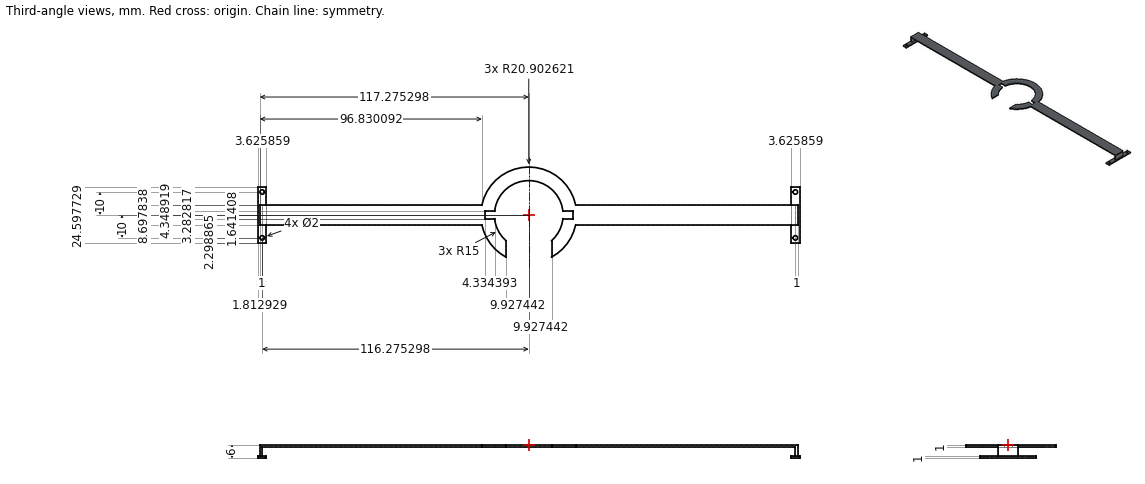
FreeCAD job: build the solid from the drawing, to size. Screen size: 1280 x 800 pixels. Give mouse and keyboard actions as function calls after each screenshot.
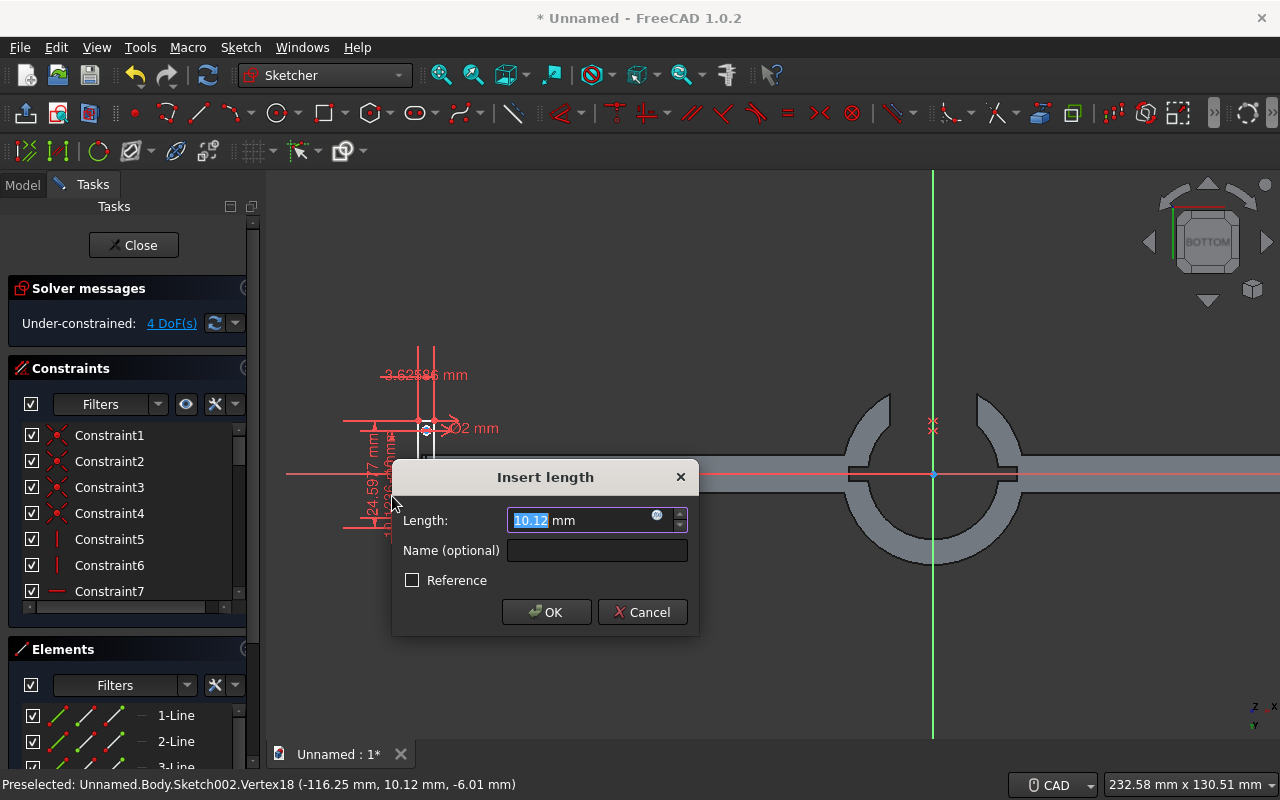
text(10)
key(Return)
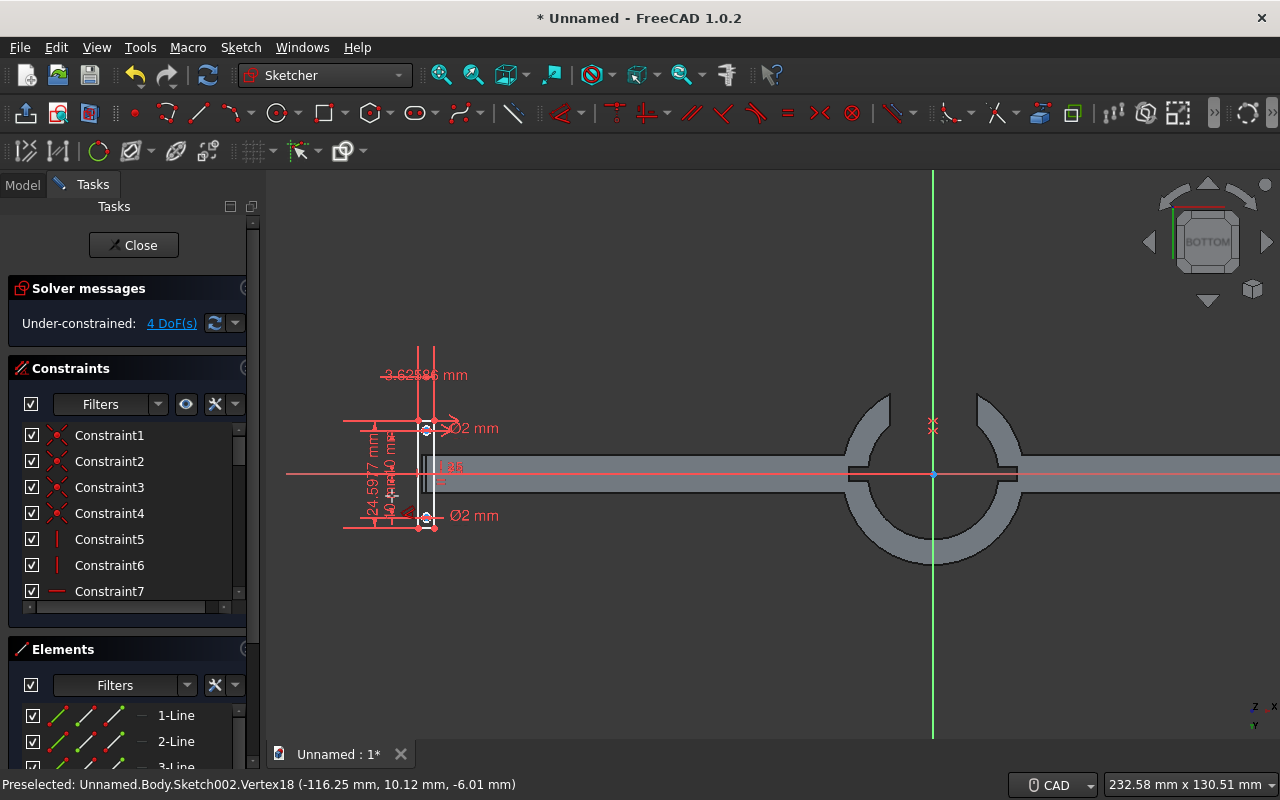
scroll(426, 431, down, 3)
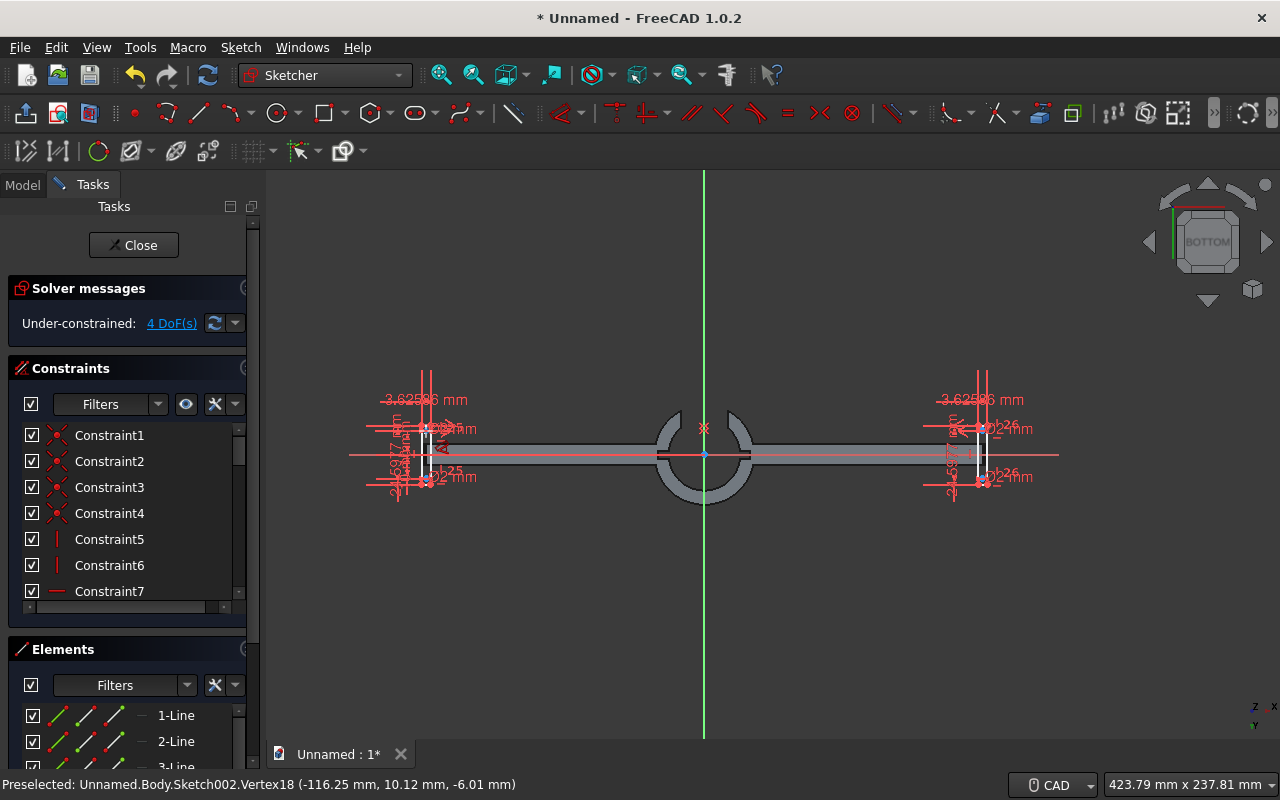
scroll(983, 479, up, 3)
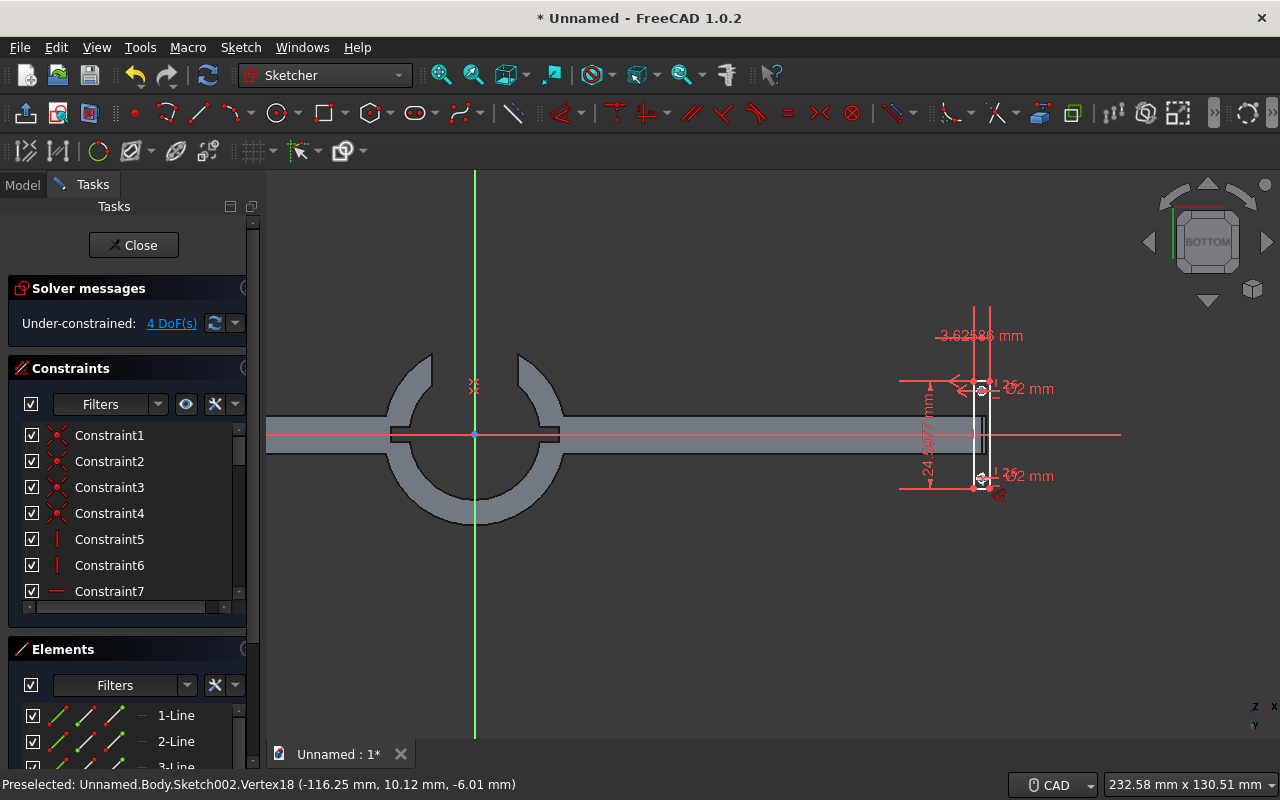
click(982, 478)
click(1016, 456)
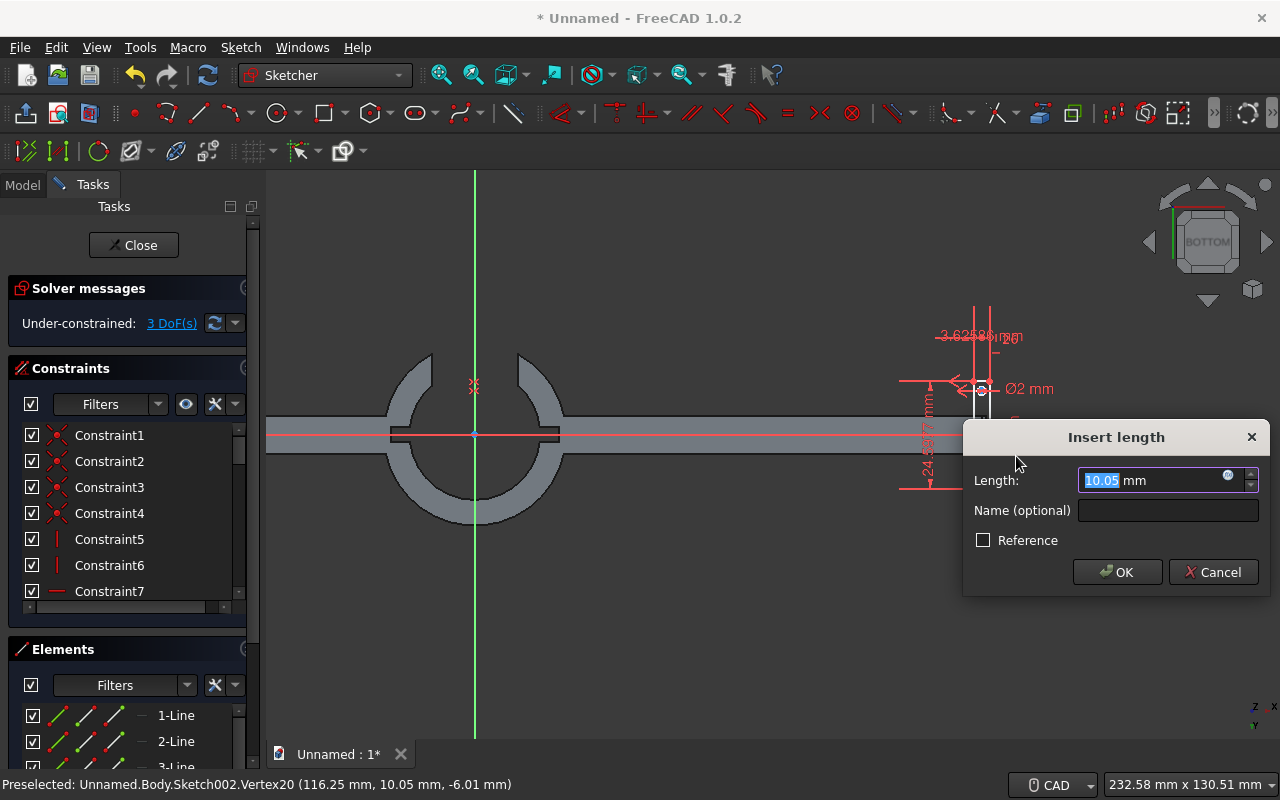
text(10)
key(Return)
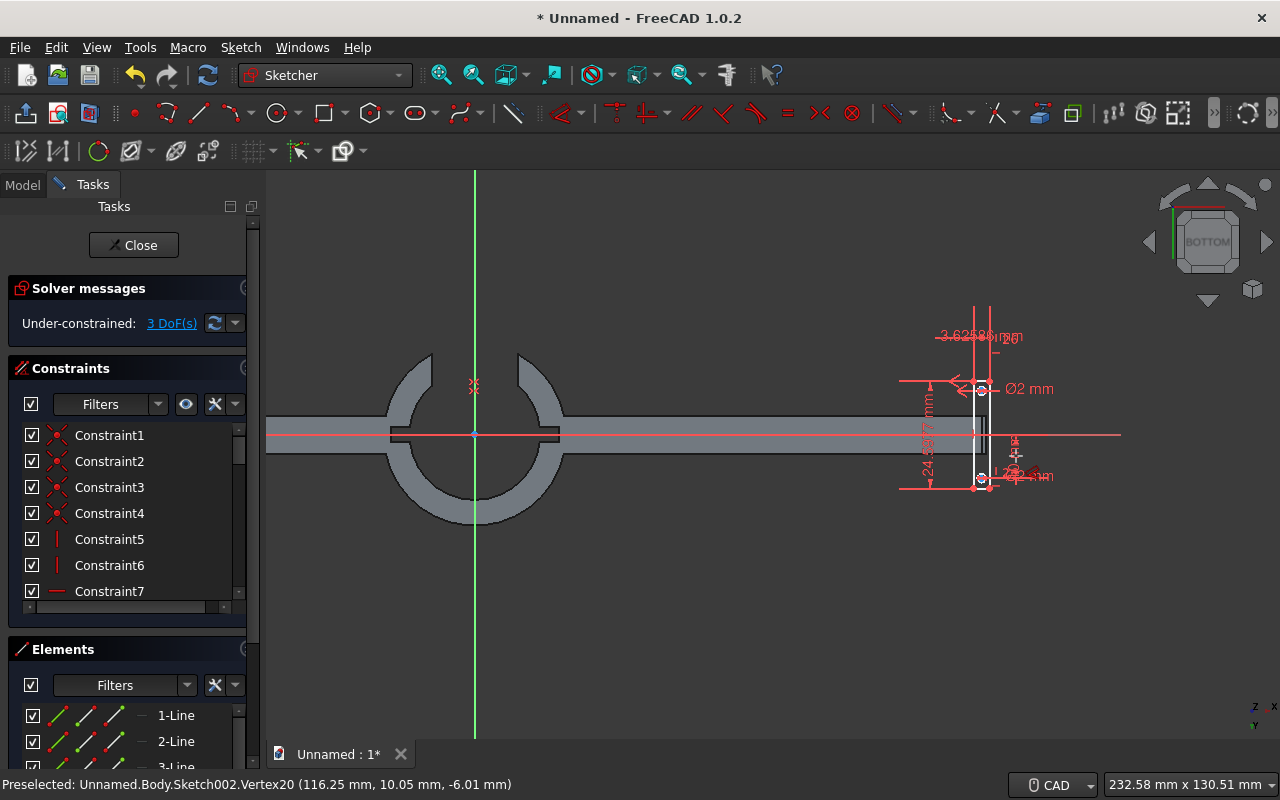
scroll(984, 479, down, 3)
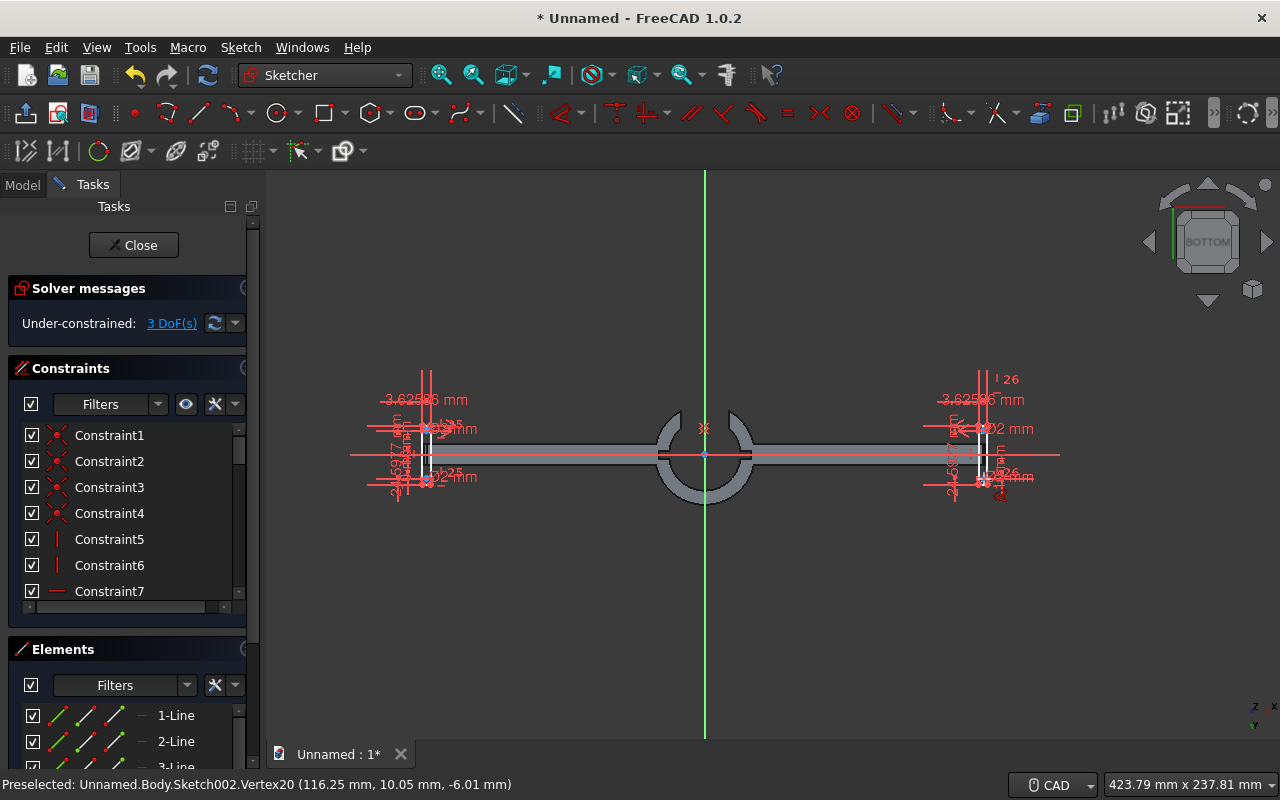
scroll(422, 426, up, 12)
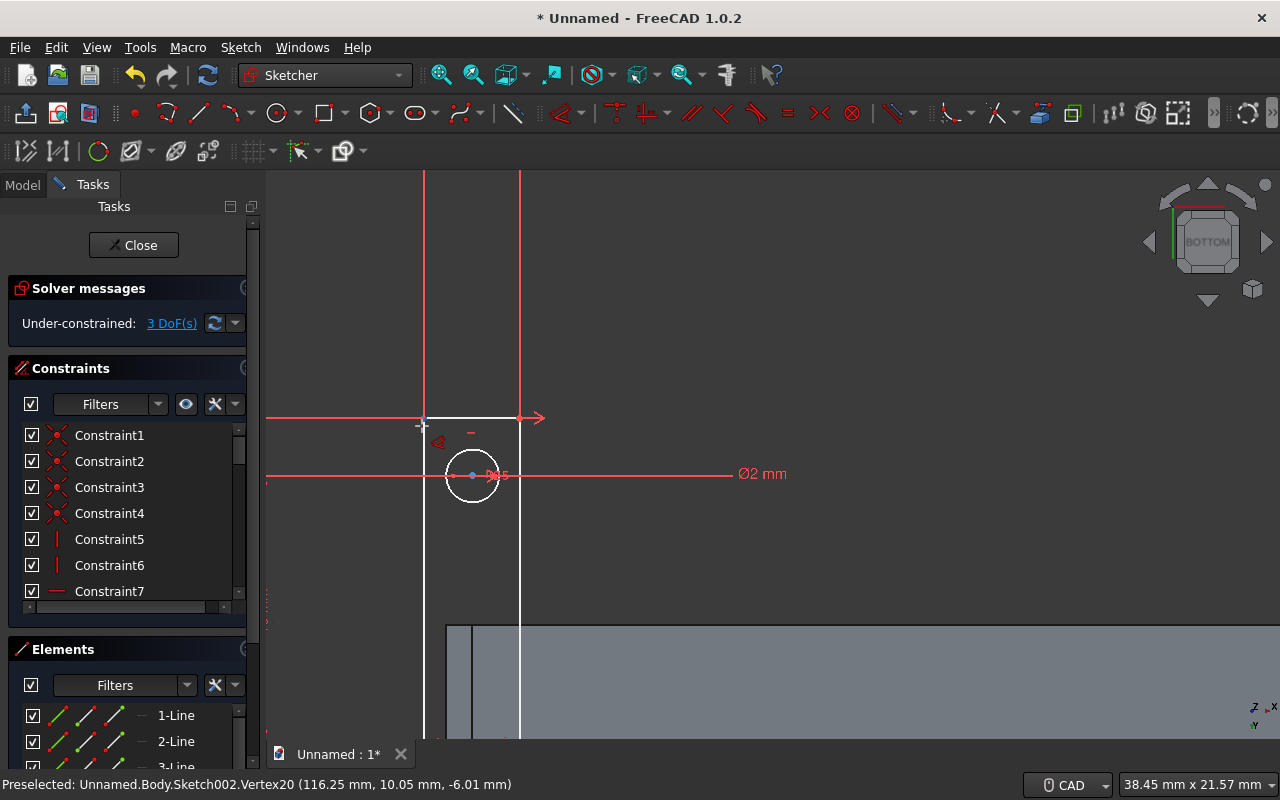
click(424, 418)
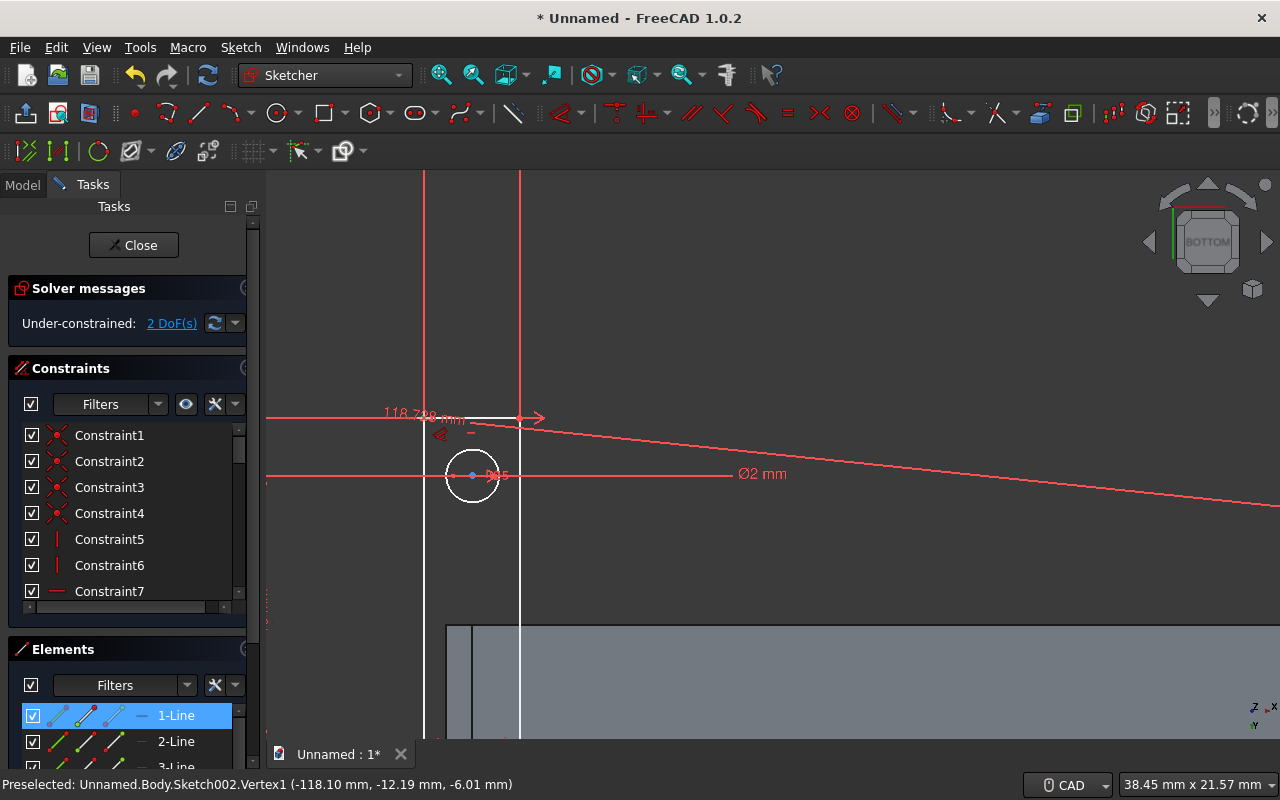
click(473, 476)
click(448, 384)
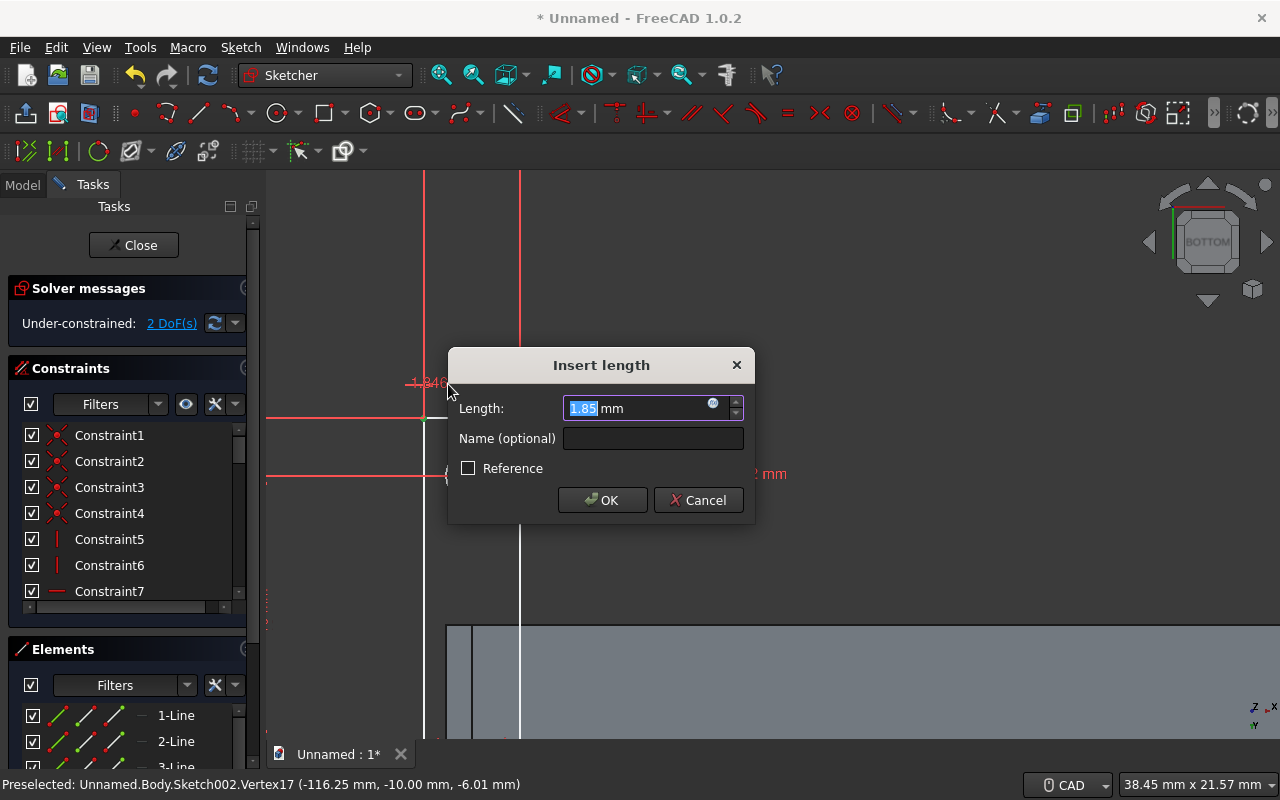
text(1.812929)
key(Return)